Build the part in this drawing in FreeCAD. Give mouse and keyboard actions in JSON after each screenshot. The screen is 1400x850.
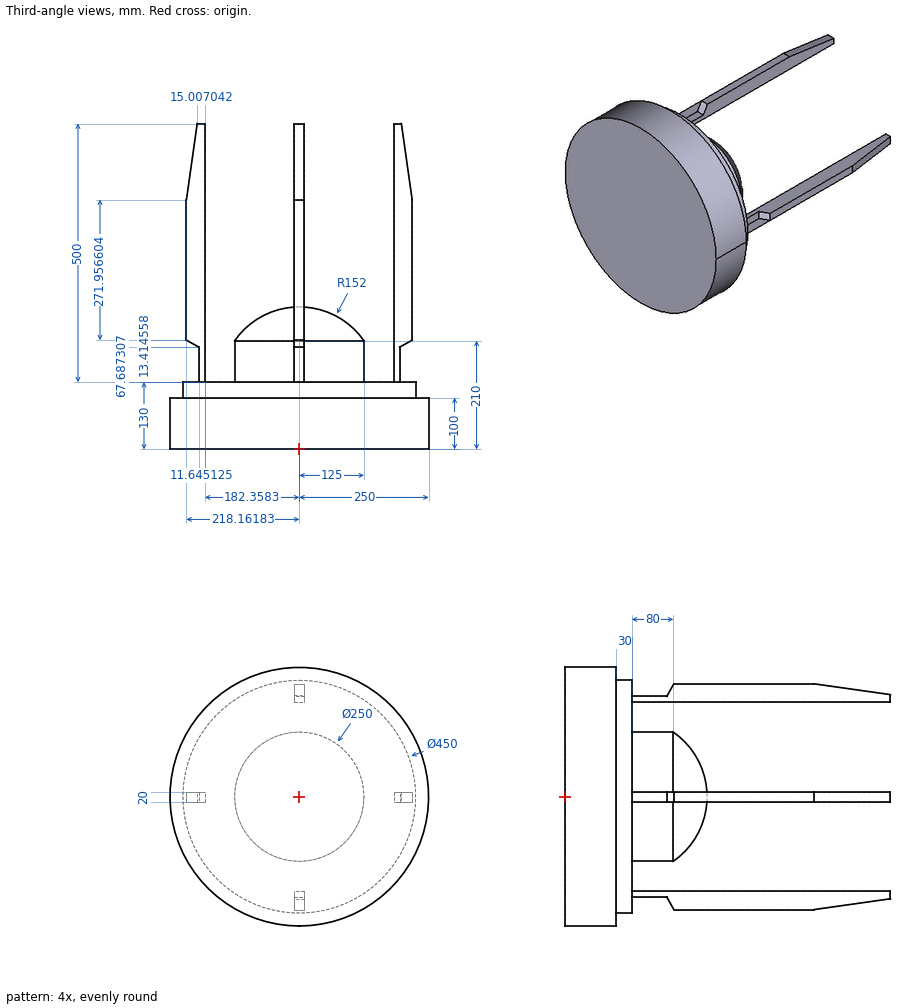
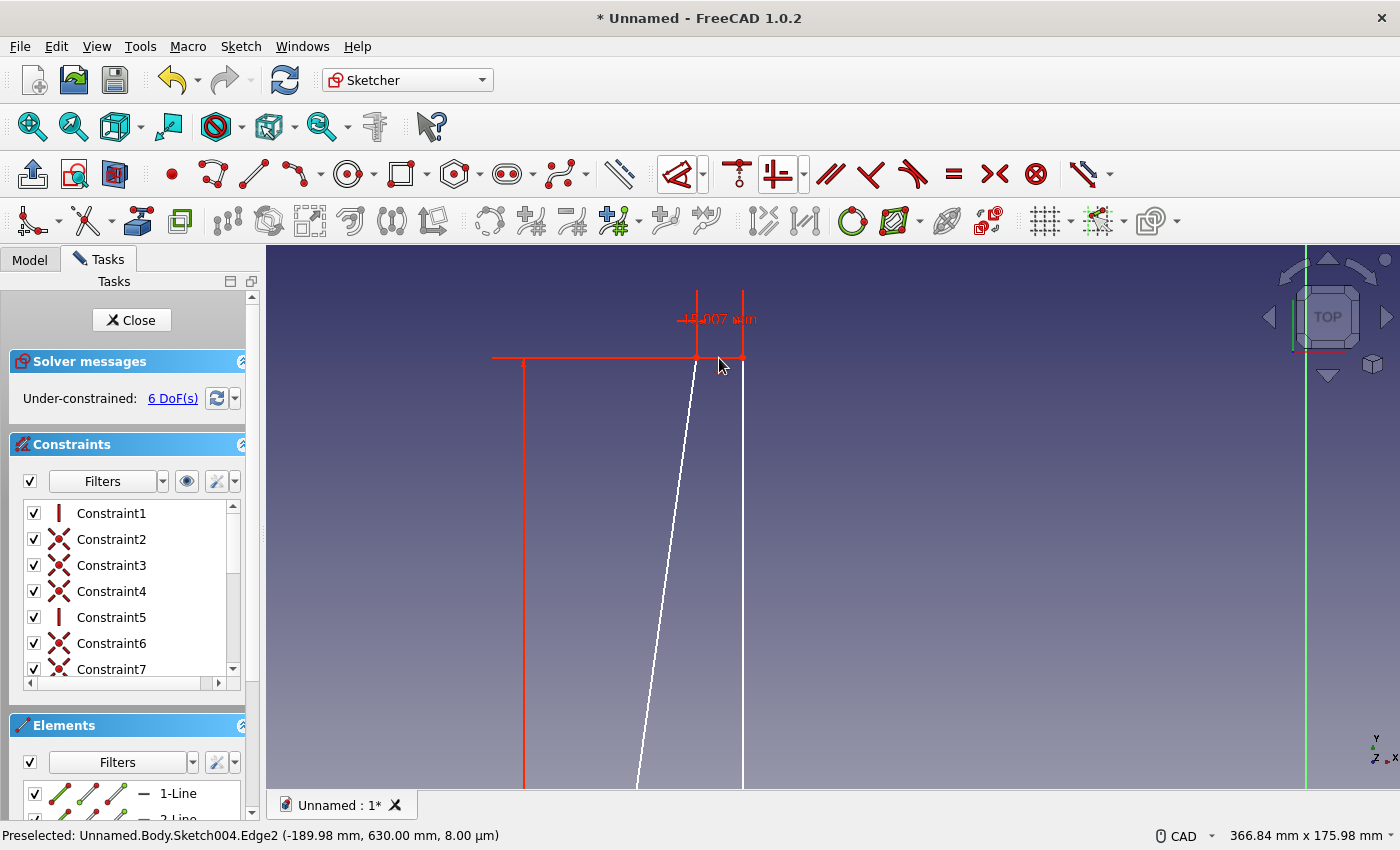
{"action": "scroll", "coordinate": [724, 356], "scroll_direction": "down", "scroll_amount": 9}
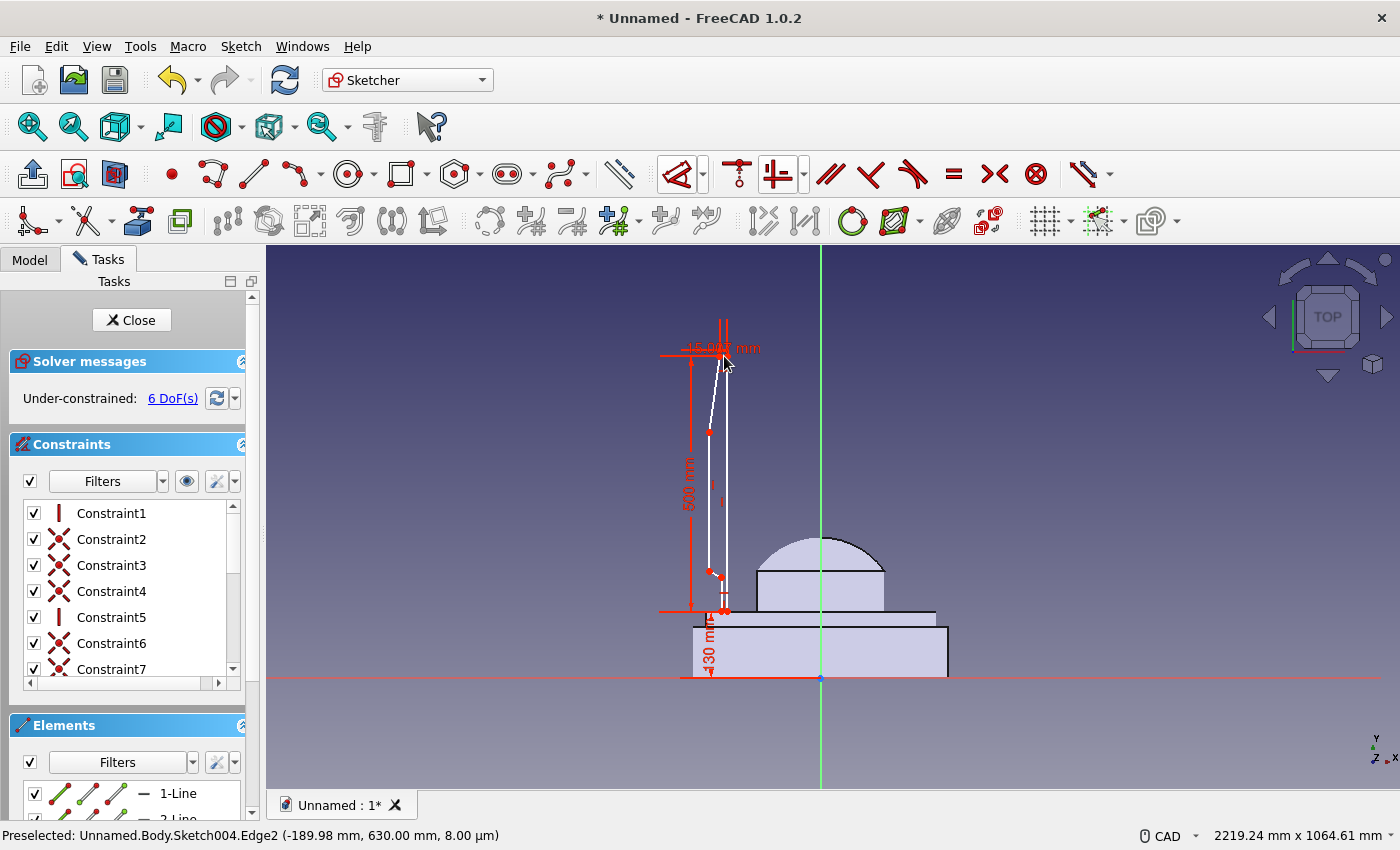
{"action": "scroll", "coordinate": [722, 588], "scroll_direction": "up", "scroll_amount": 5}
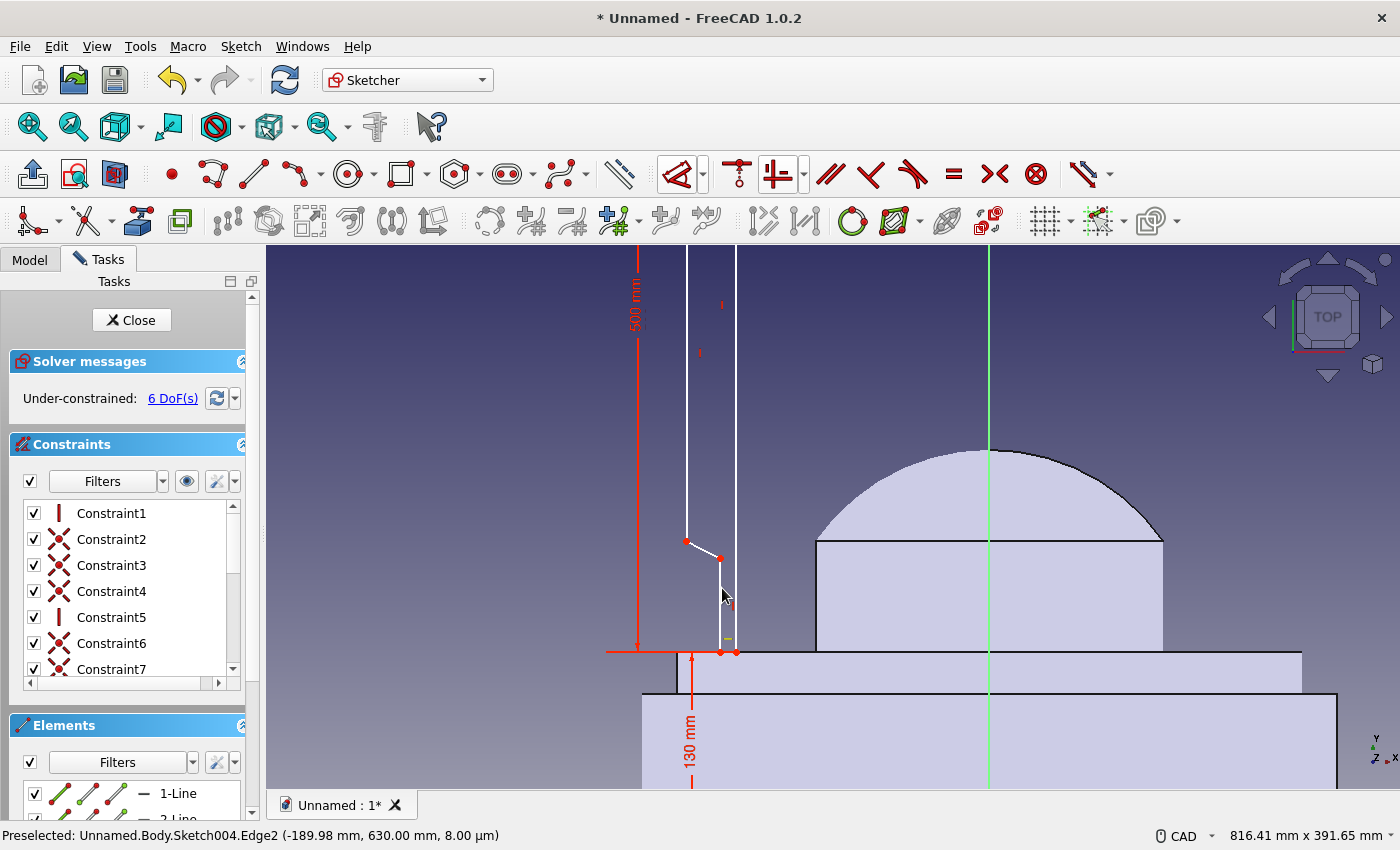
{"action": "left_click", "coordinate": [720, 587]}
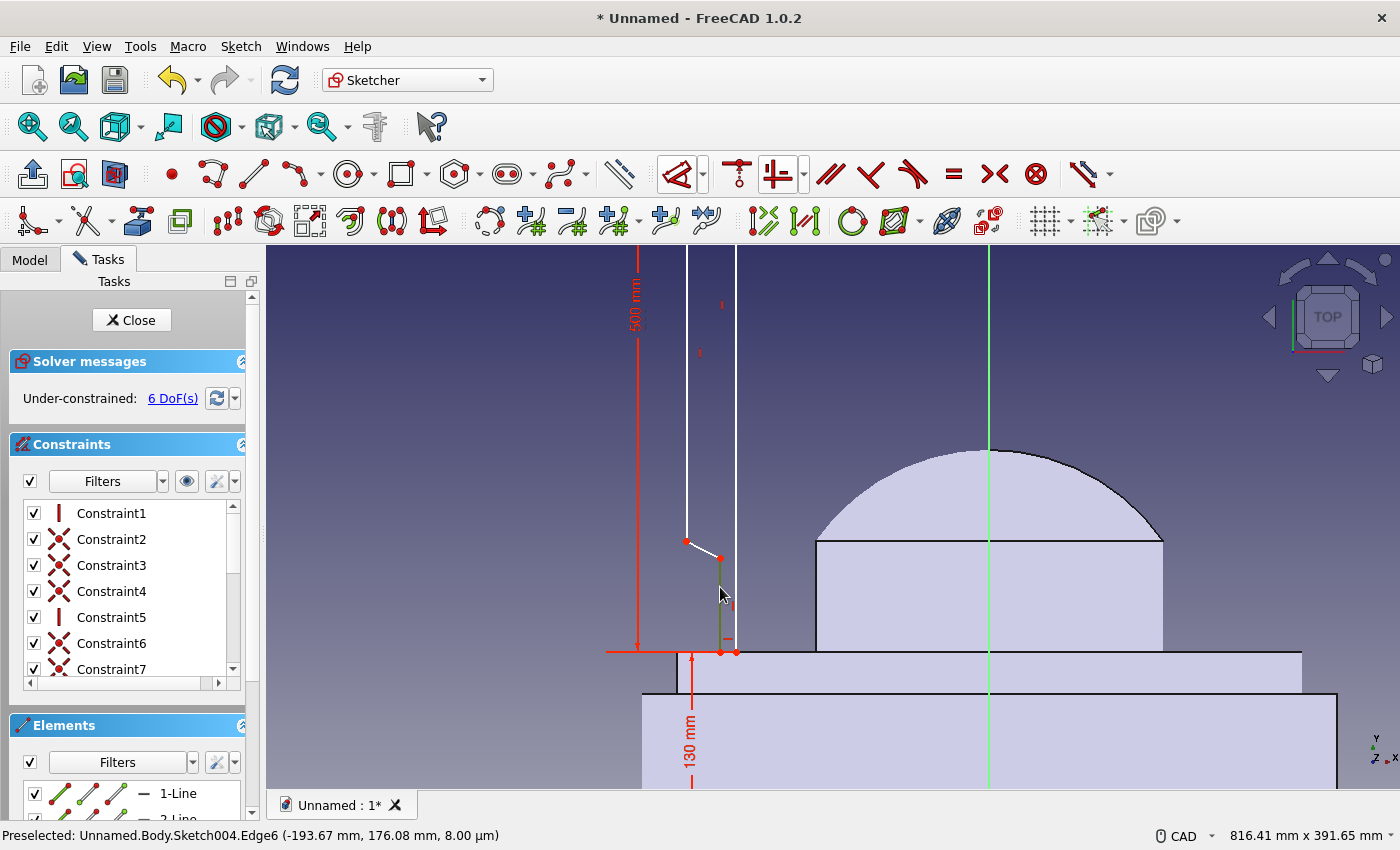
{"action": "key", "text": "i"}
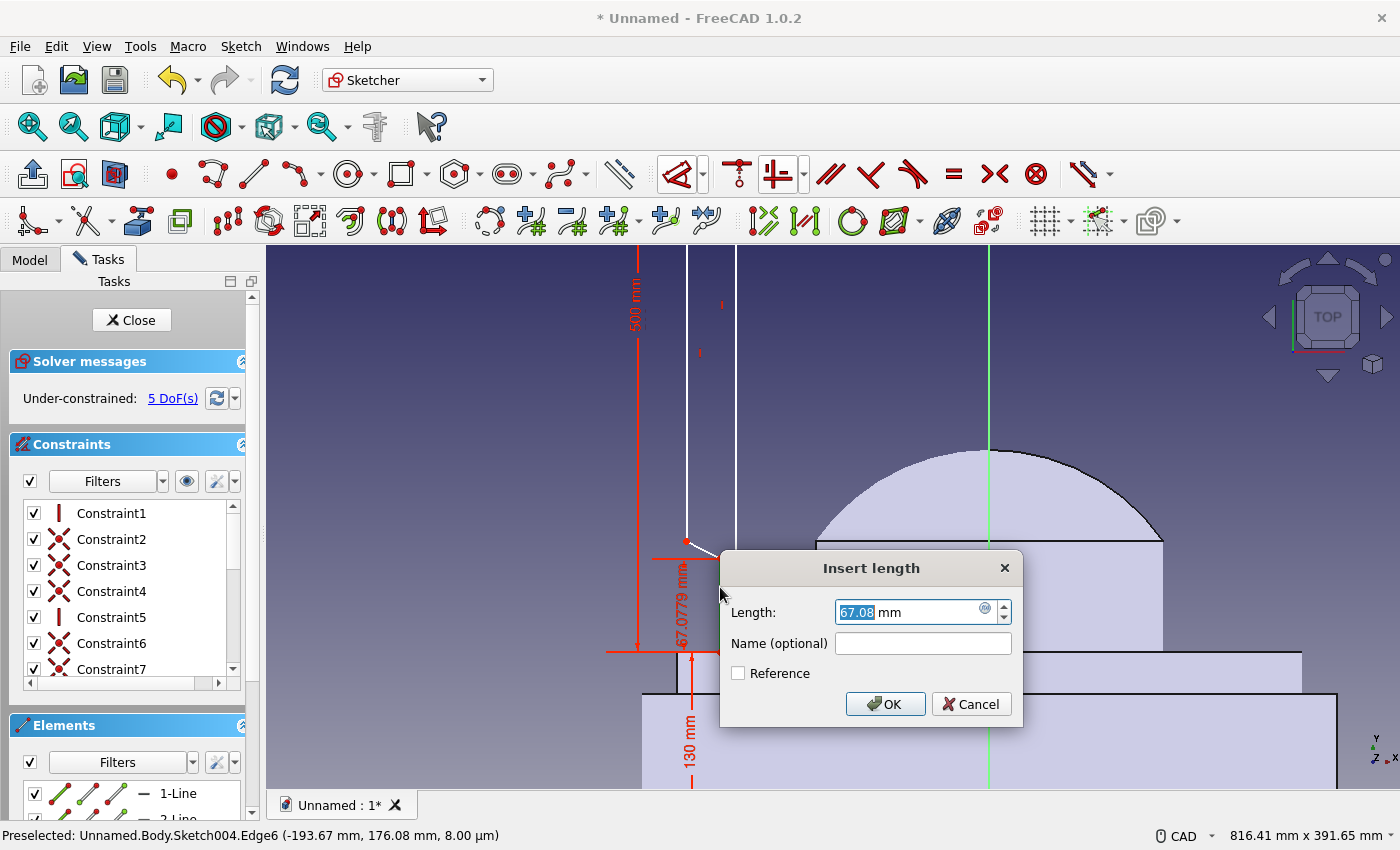
{"action": "type", "text": "67.687307"}
{"action": "key", "text": "Return"}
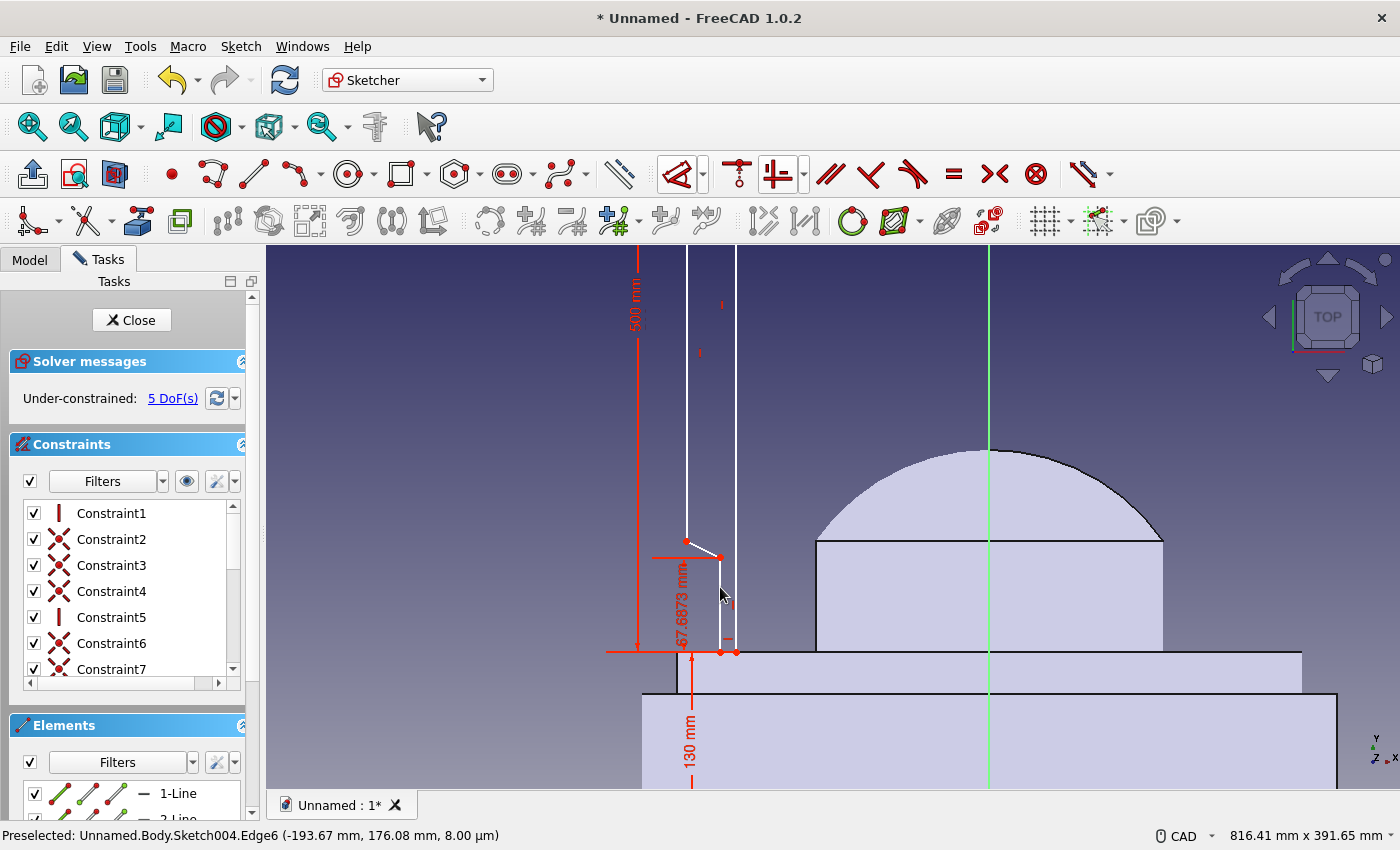
{"action": "scroll", "coordinate": [728, 652], "scroll_direction": "up", "scroll_amount": 5}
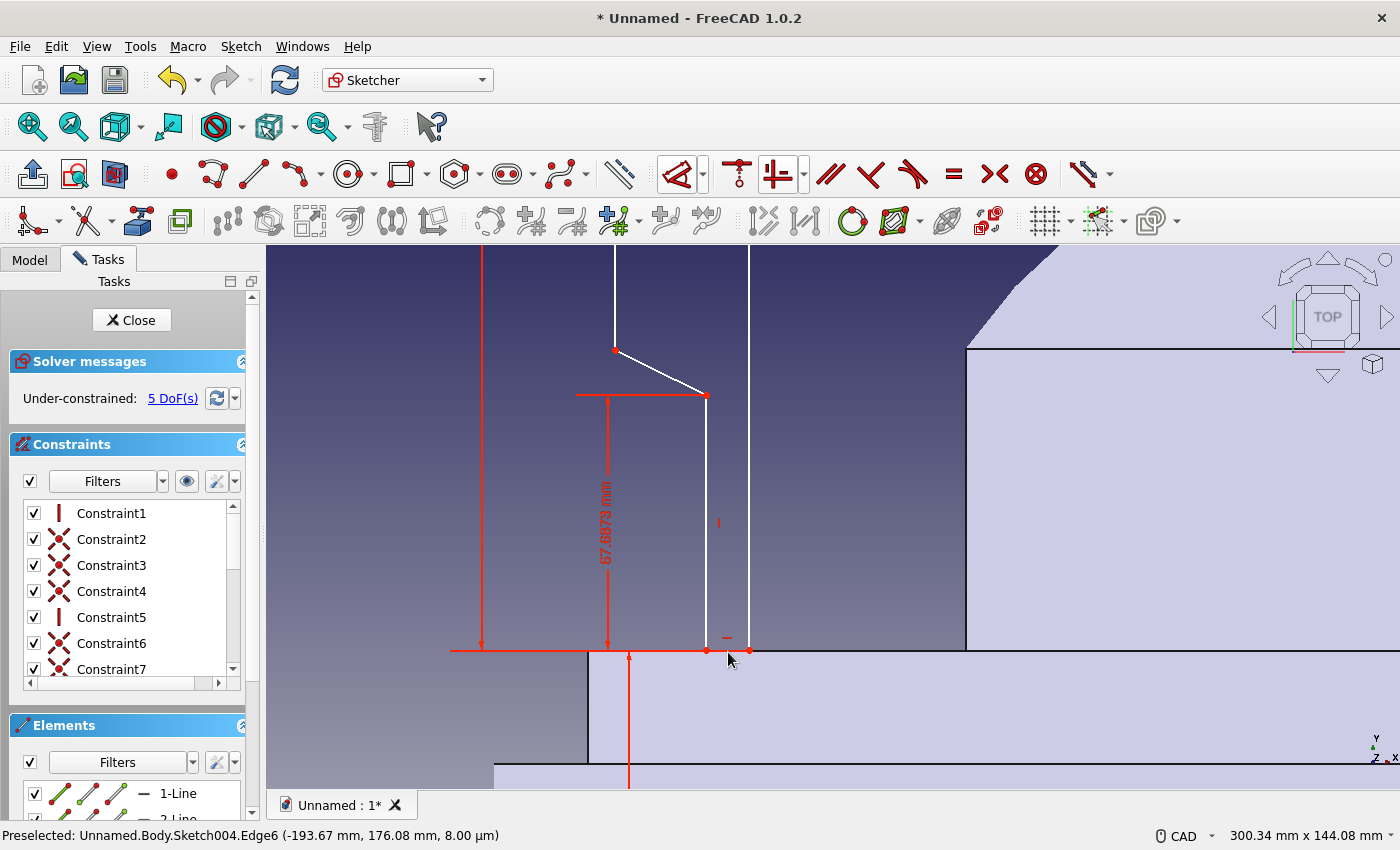
{"action": "left_click", "coordinate": [728, 651]}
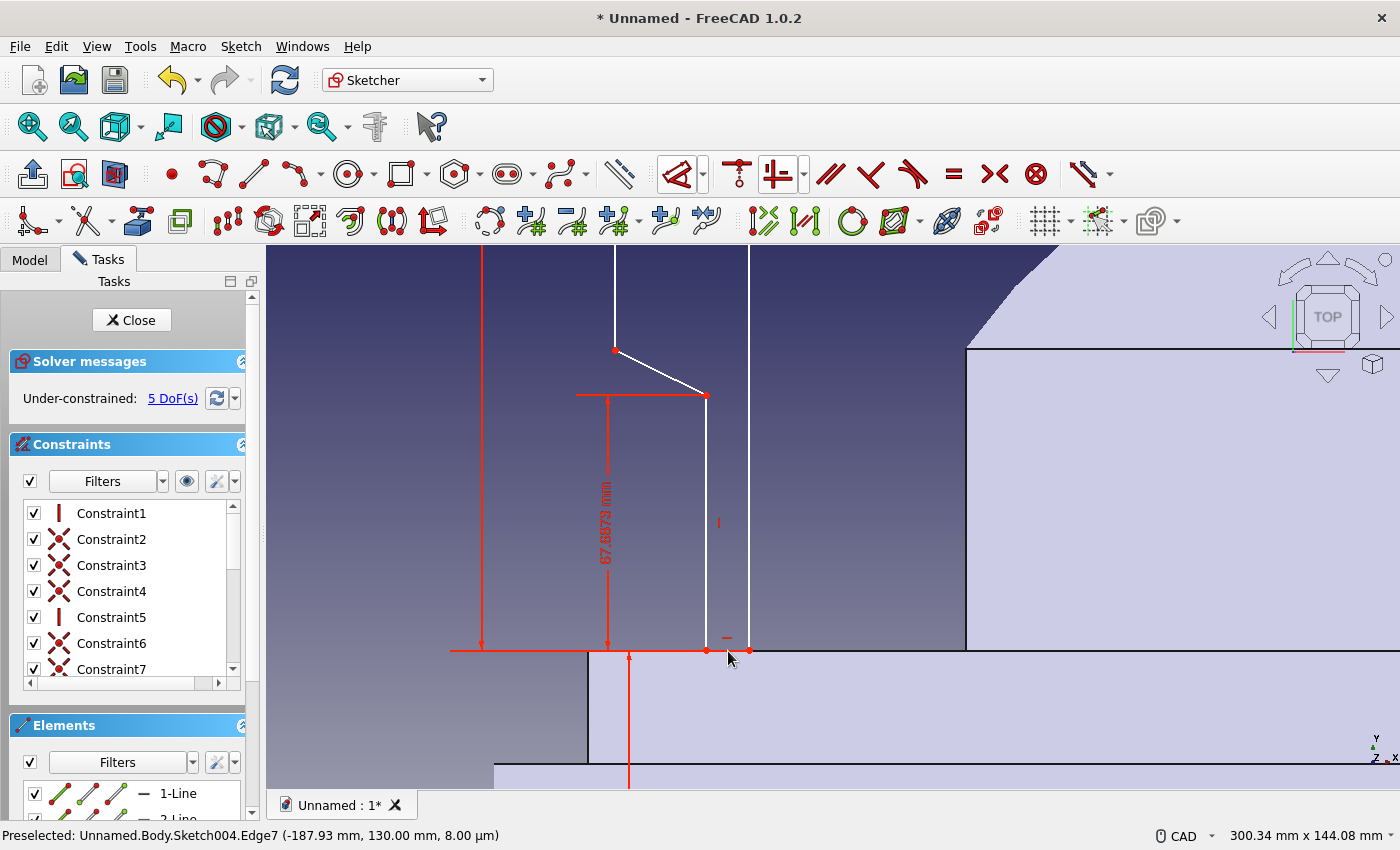
{"action": "key", "text": "l"}